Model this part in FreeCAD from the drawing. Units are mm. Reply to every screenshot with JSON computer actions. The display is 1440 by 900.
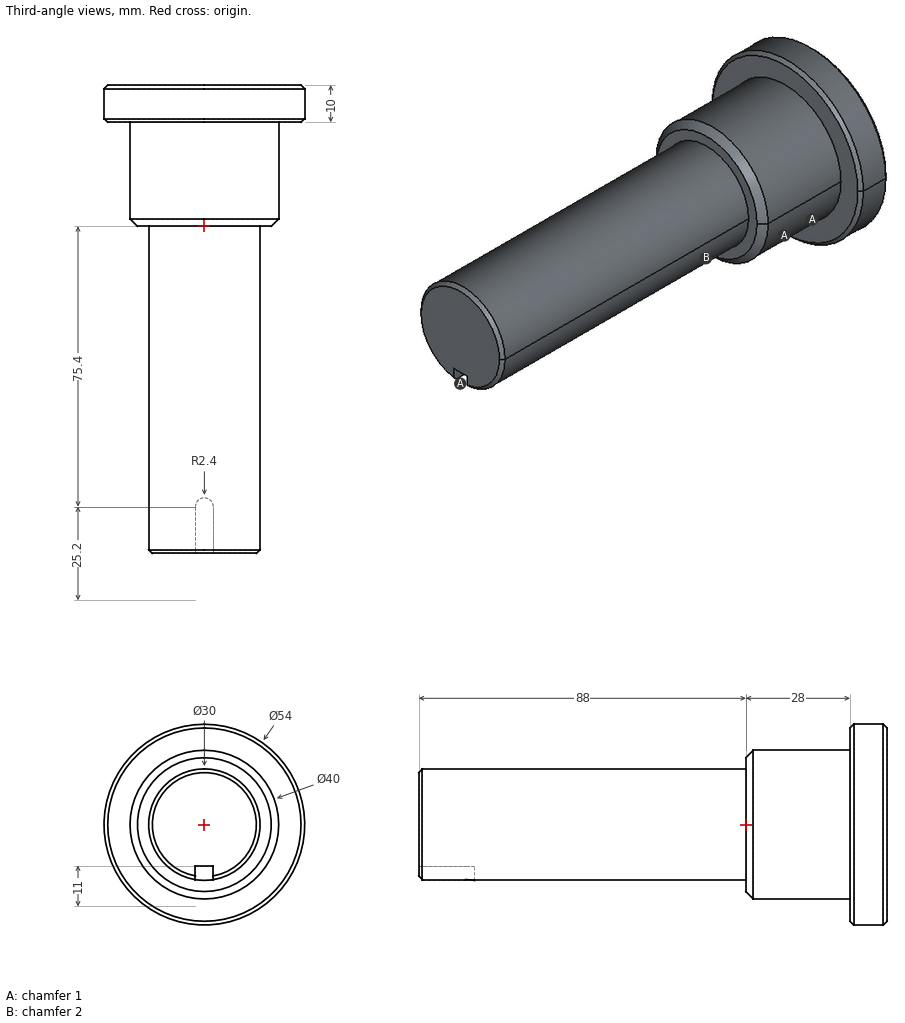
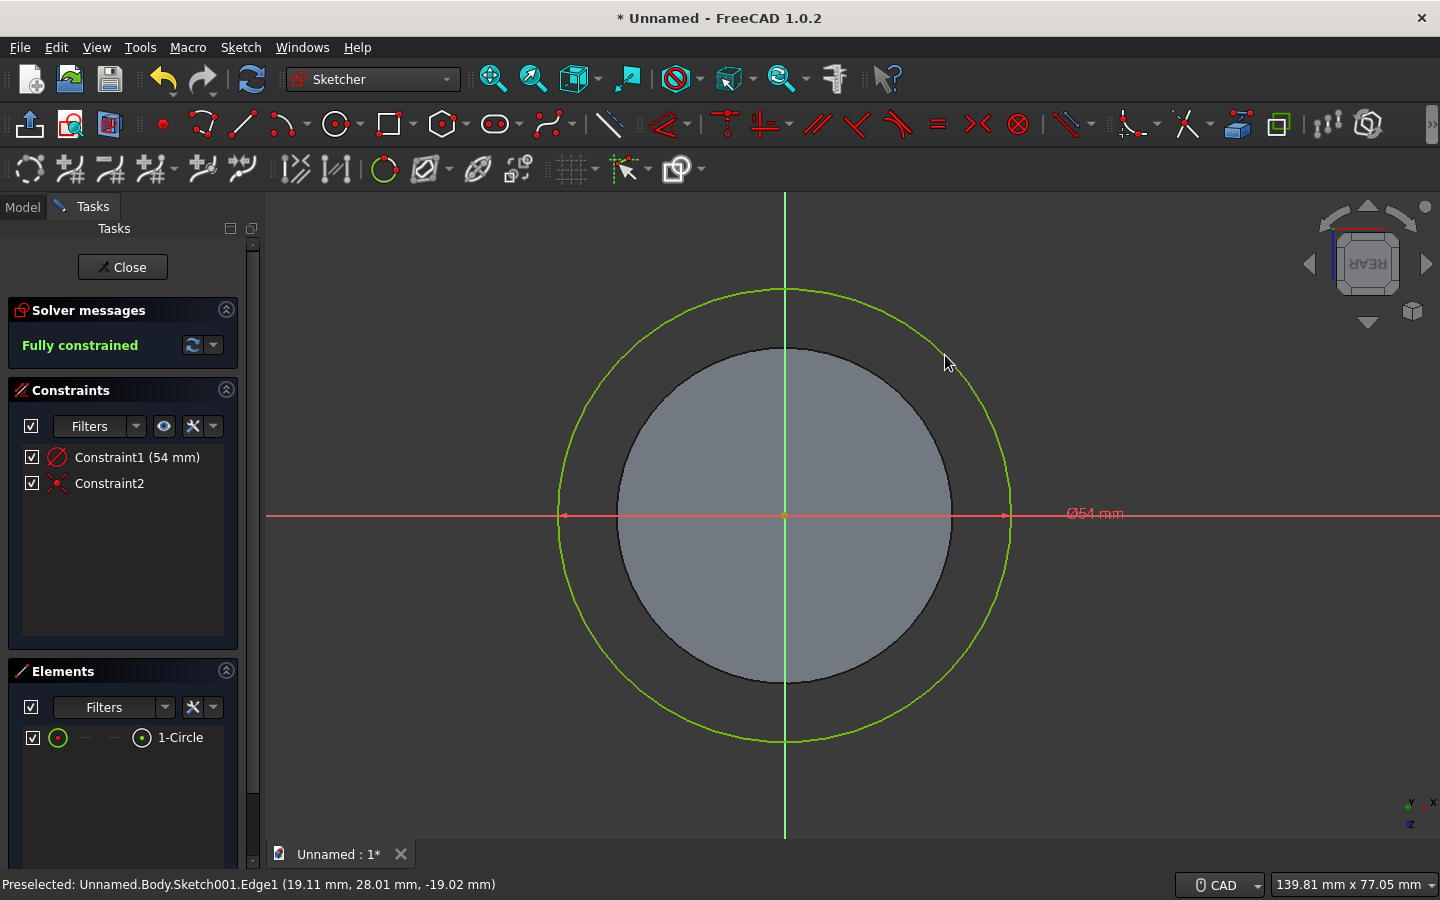
{"action": "left_click", "coordinate": [123, 267]}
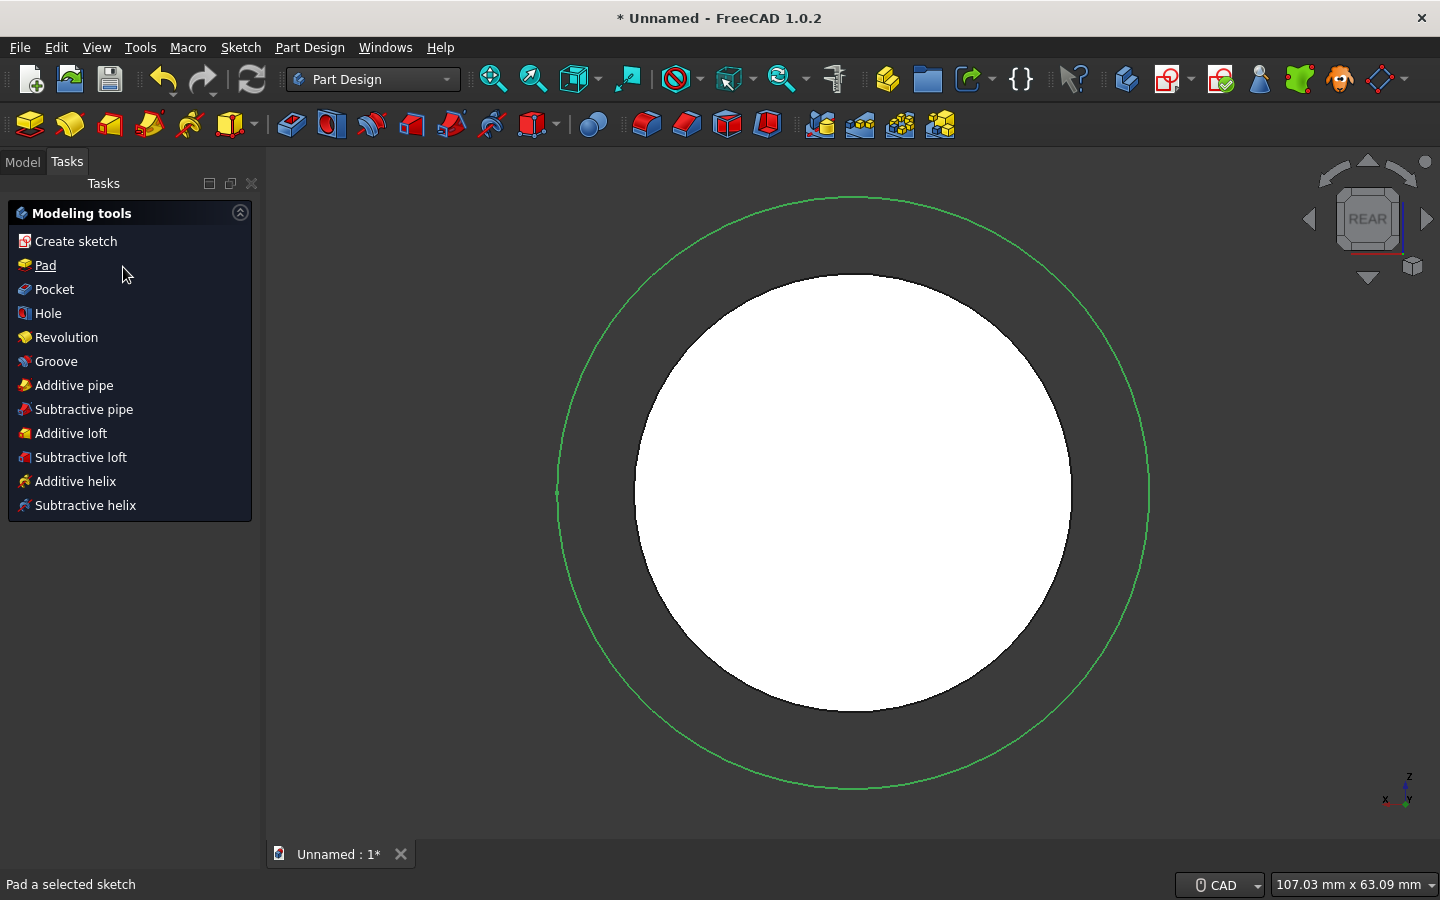
{"action": "left_click", "coordinate": [30, 124]}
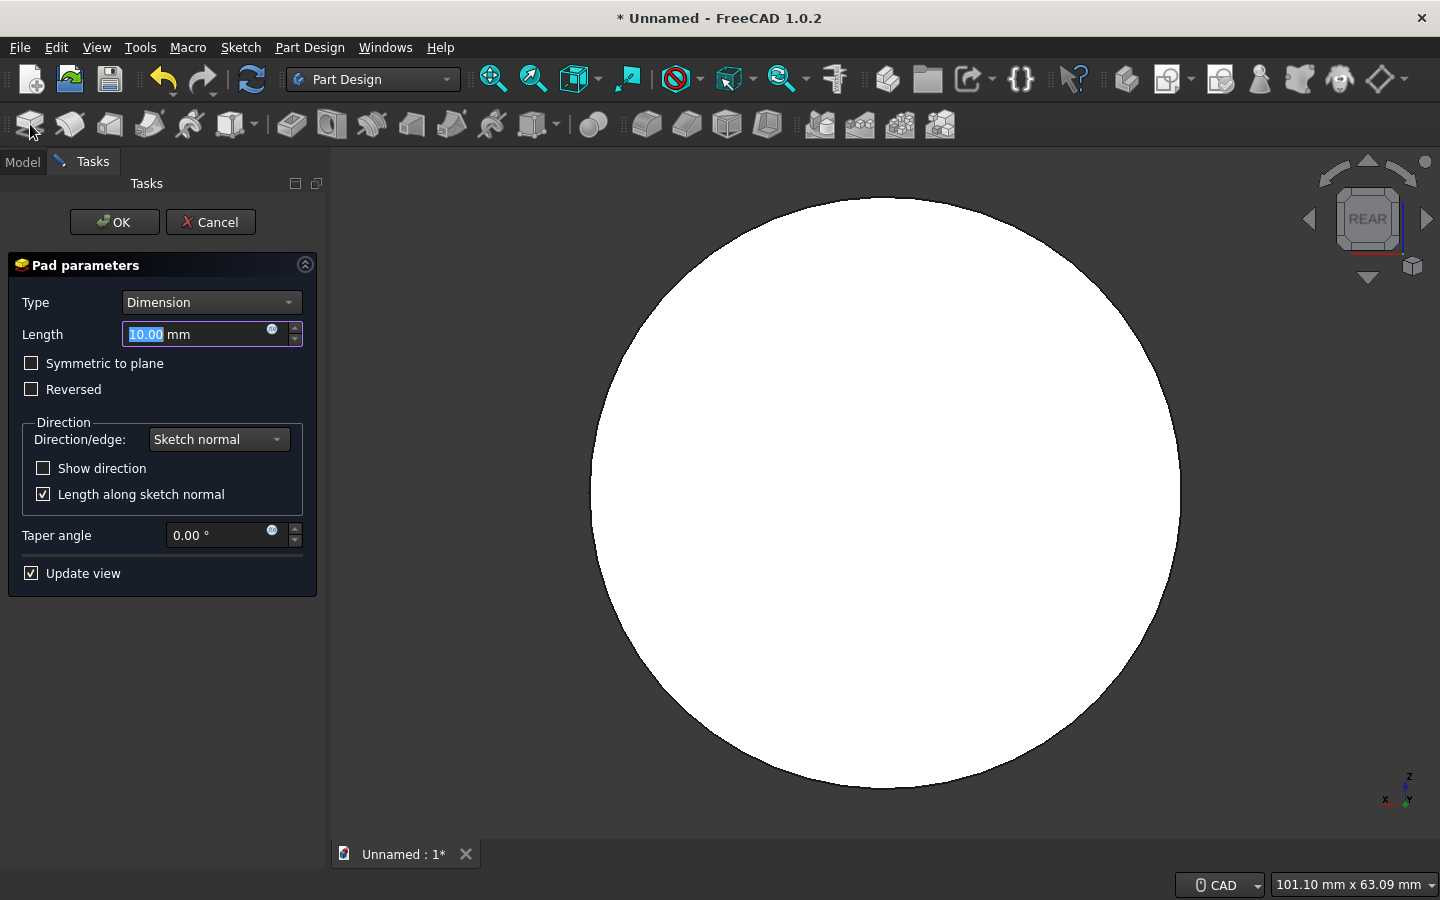
{"action": "type", "text": "10"}
{"action": "key", "text": "Tab"}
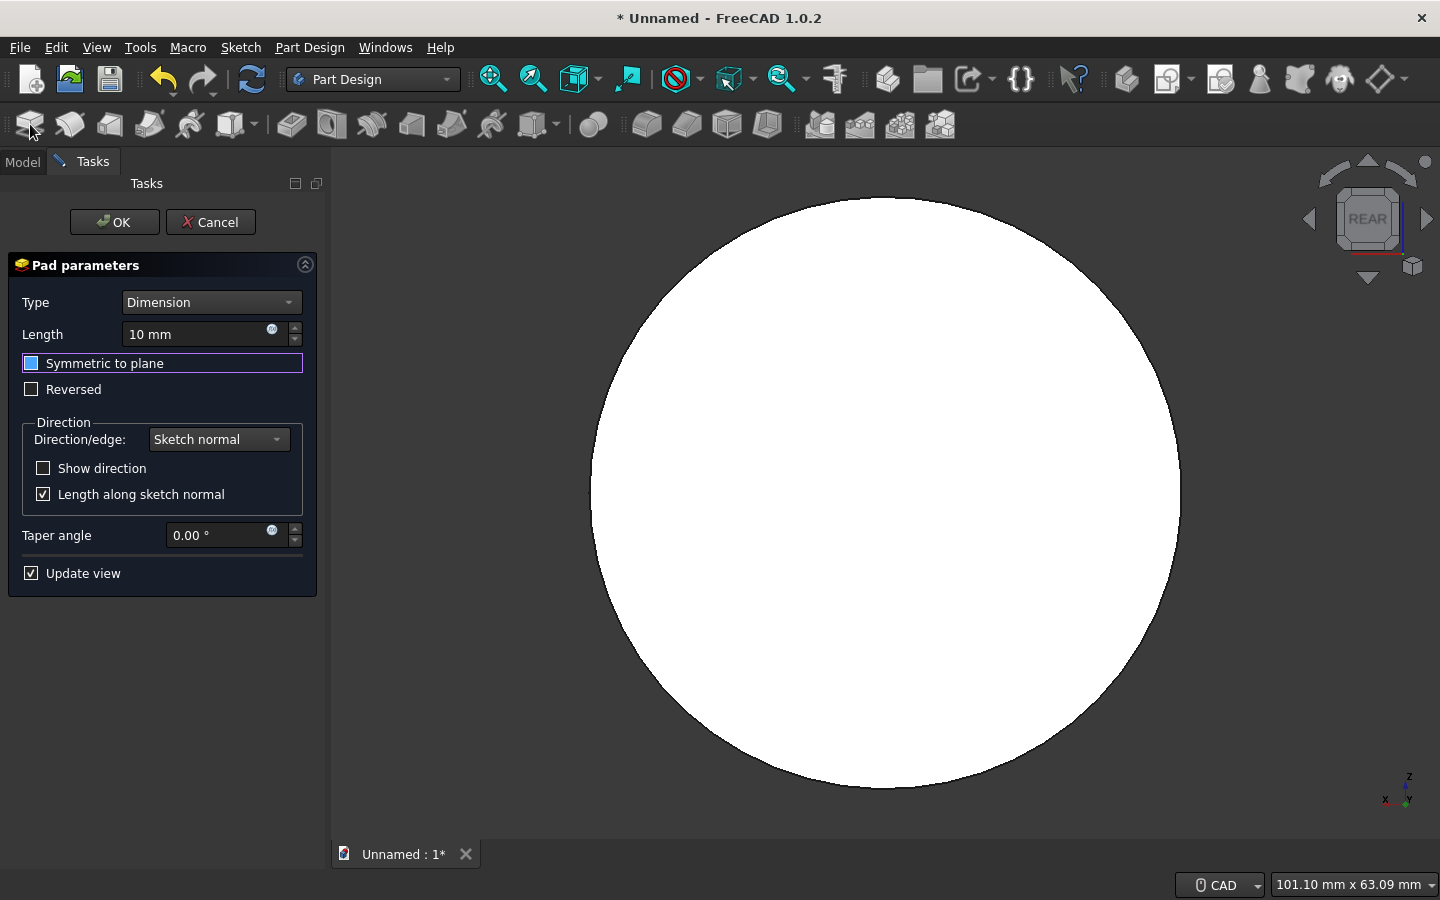
{"action": "left_click", "coordinate": [115, 222]}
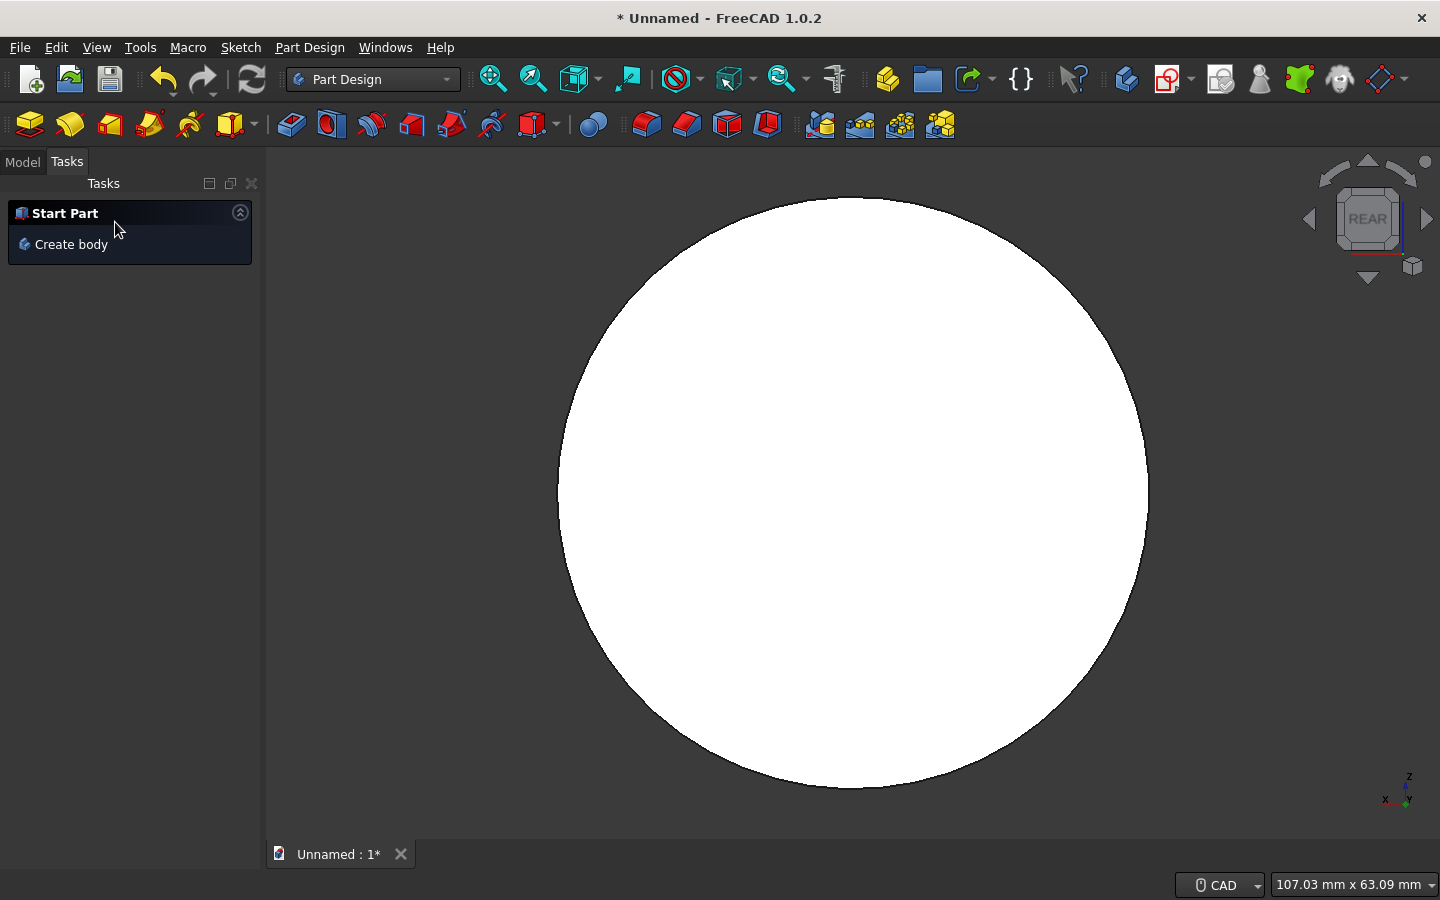
{"action": "key", "text": "0"}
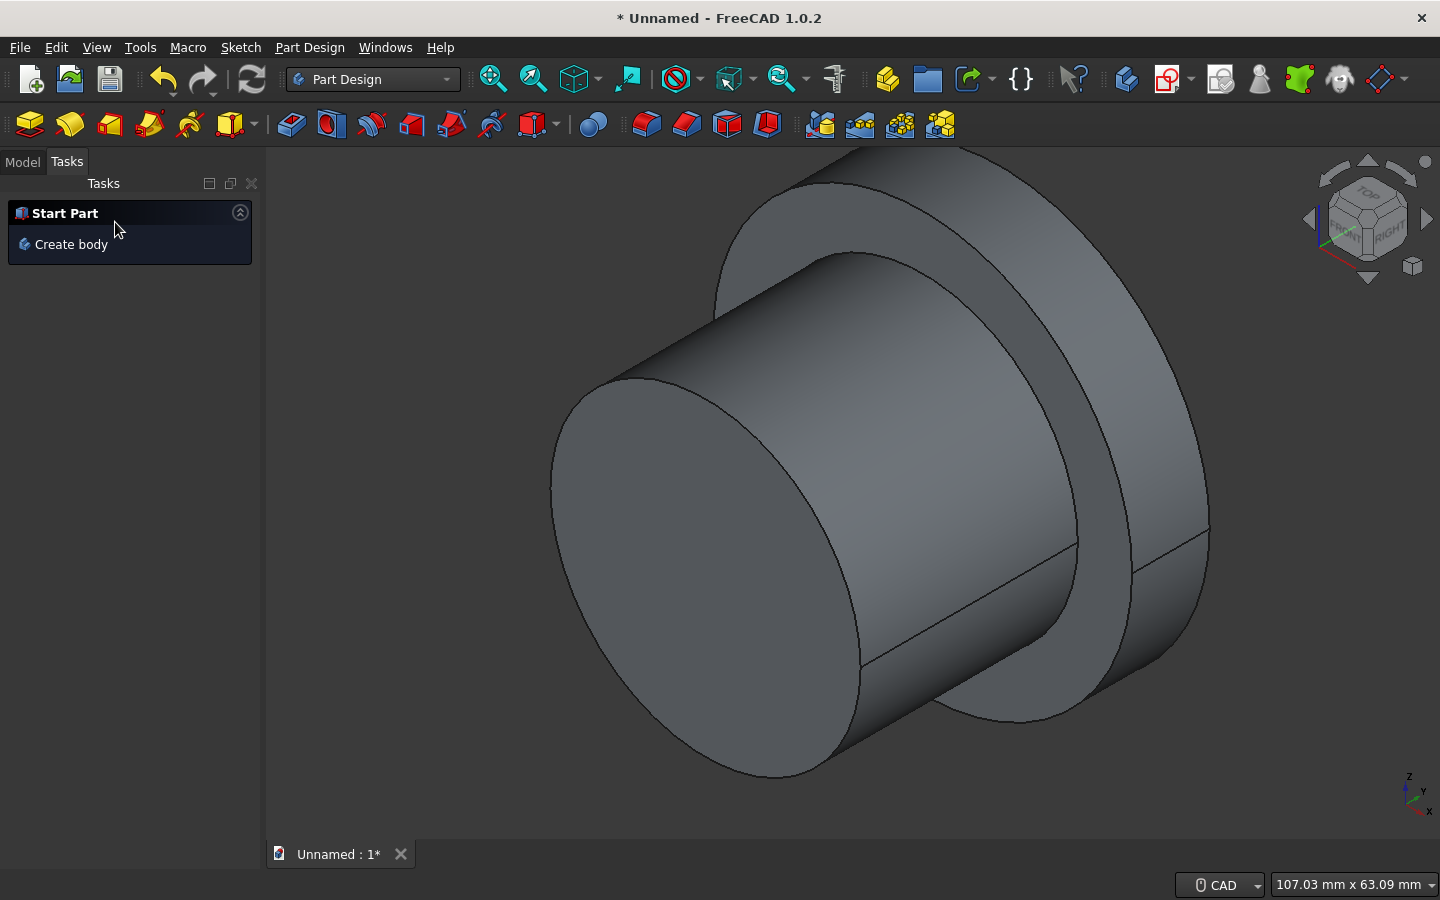
{"action": "left_click", "coordinate": [494, 80]}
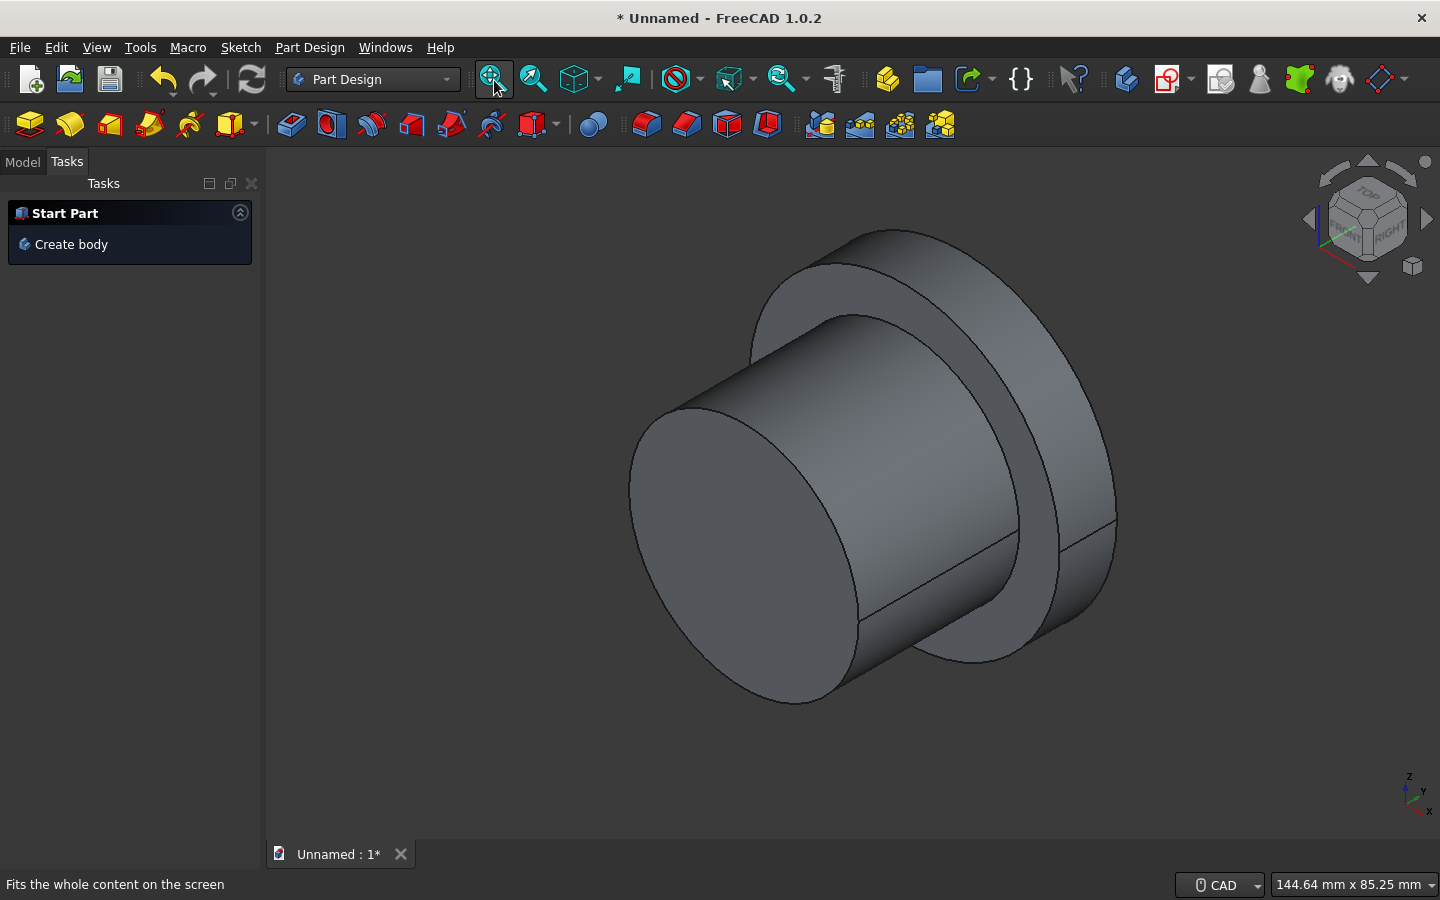
{"action": "left_click", "coordinate": [744, 555]}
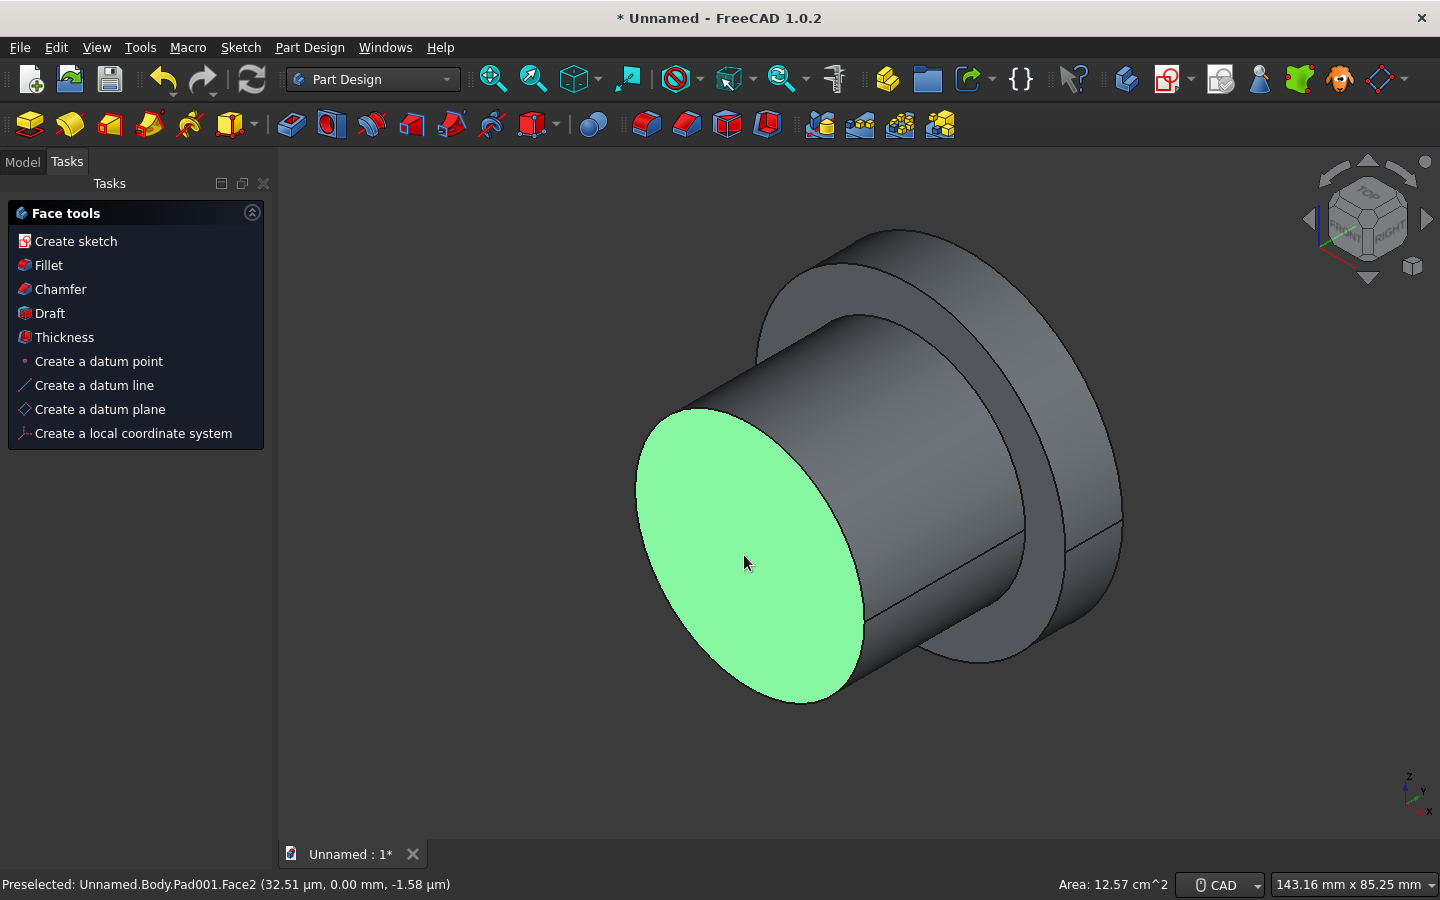
{"action": "left_click", "coordinate": [1168, 80]}